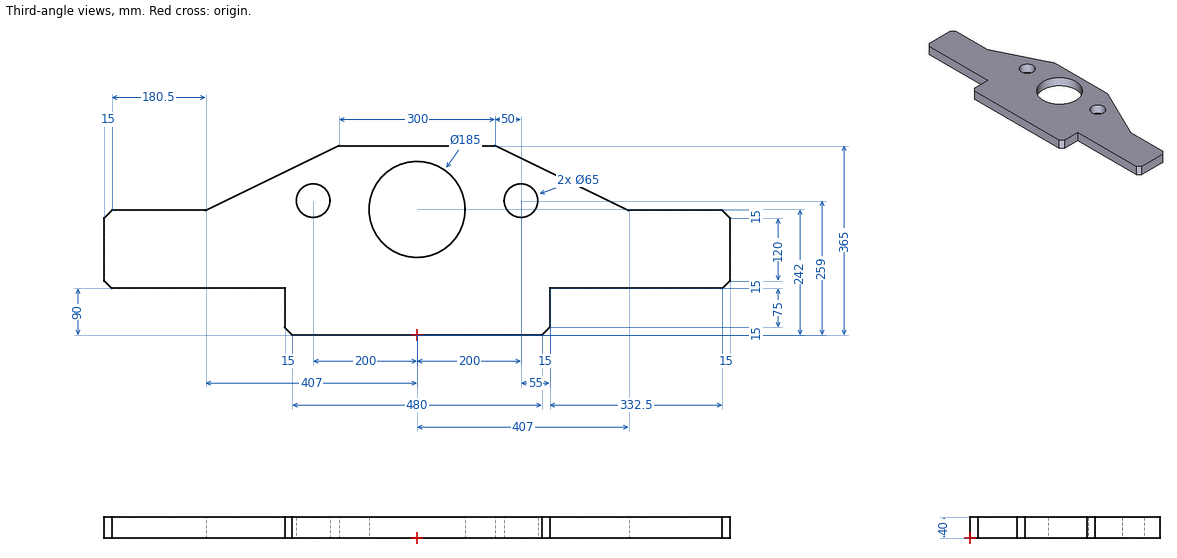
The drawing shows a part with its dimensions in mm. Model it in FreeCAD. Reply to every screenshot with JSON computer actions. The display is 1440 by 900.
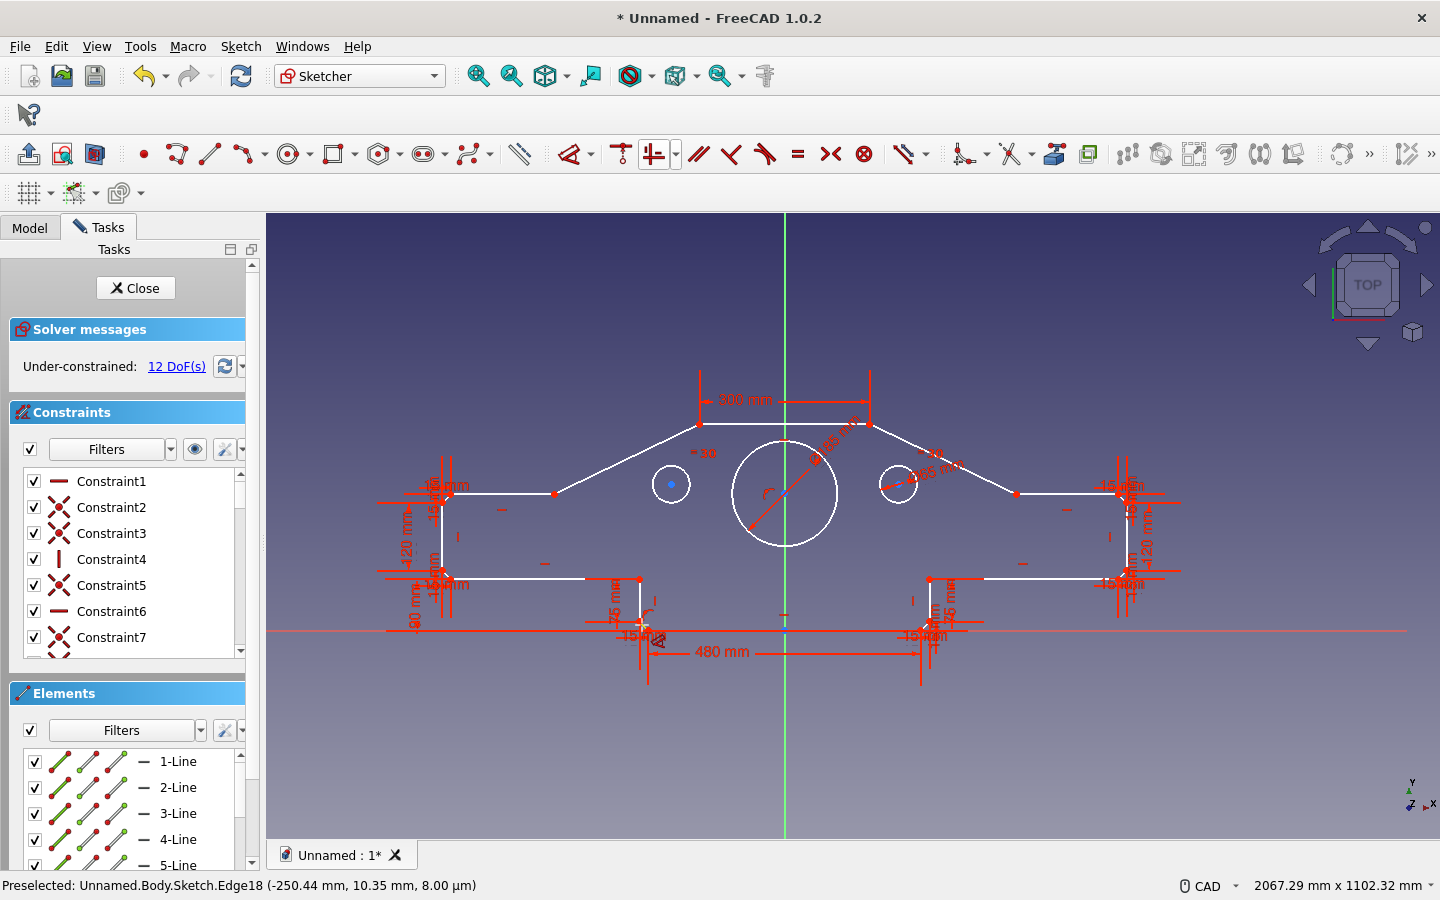
{"action": "left_click", "coordinate": [899, 484]}
{"action": "left_click", "coordinate": [842, 665]}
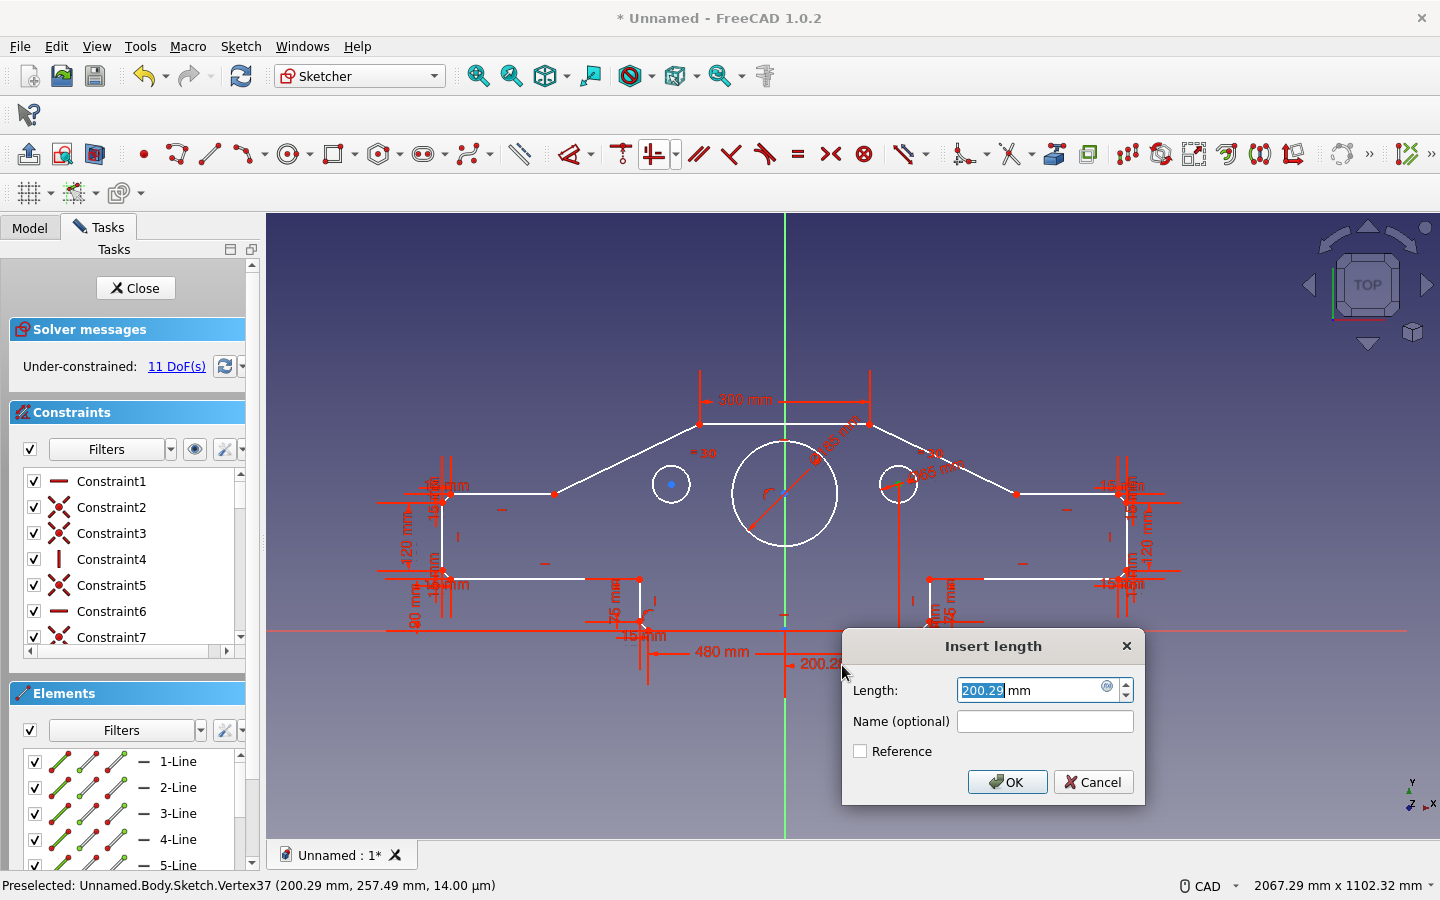
{"action": "type", "text": "200"}
{"action": "key", "text": "Return"}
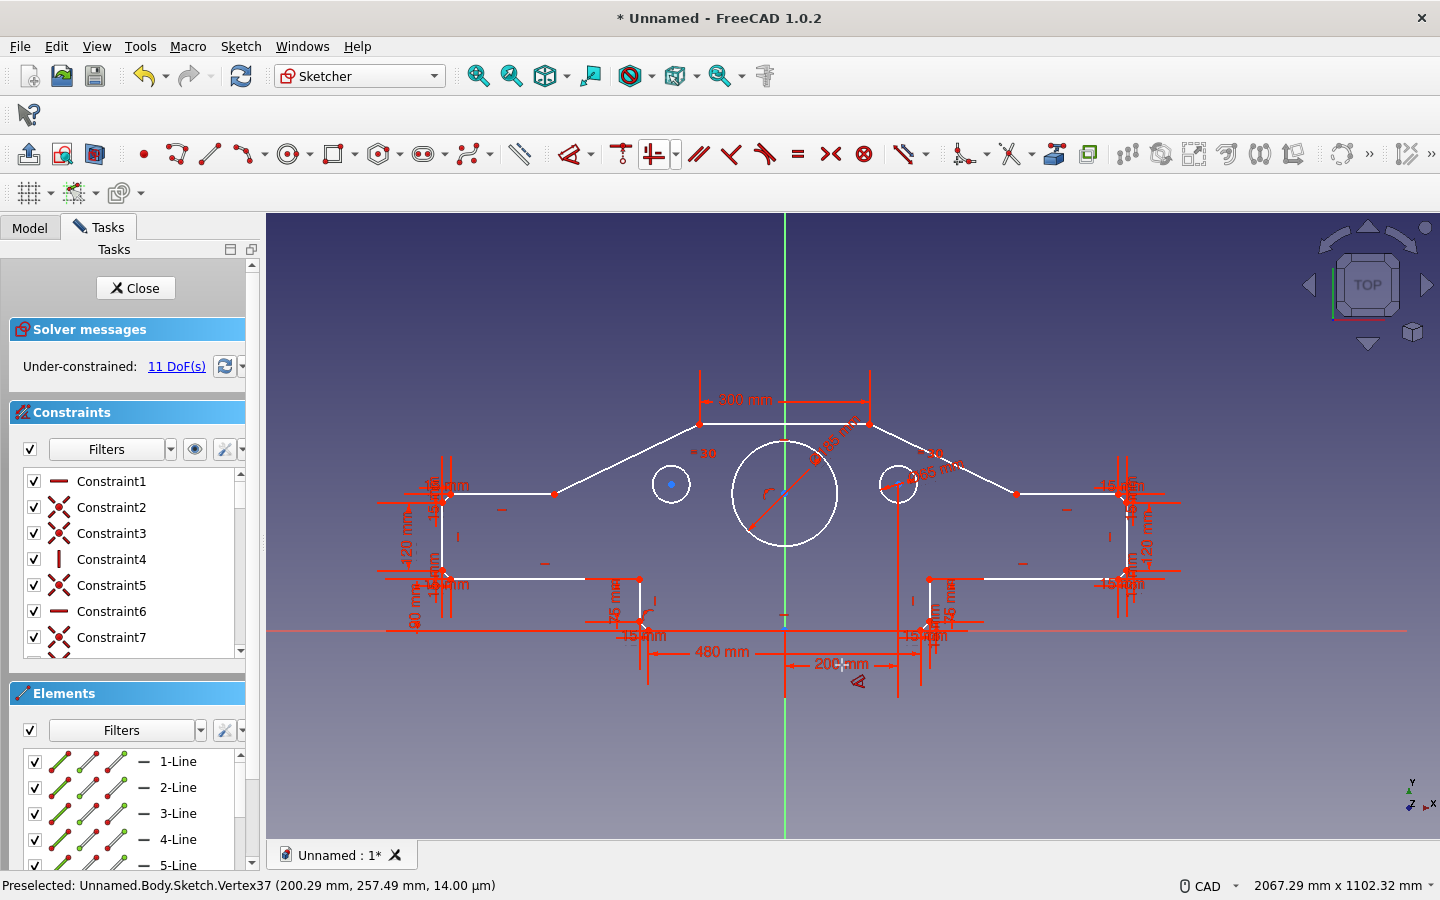
{"action": "left_click", "coordinate": [898, 484]}
{"action": "left_click", "coordinate": [932, 557]}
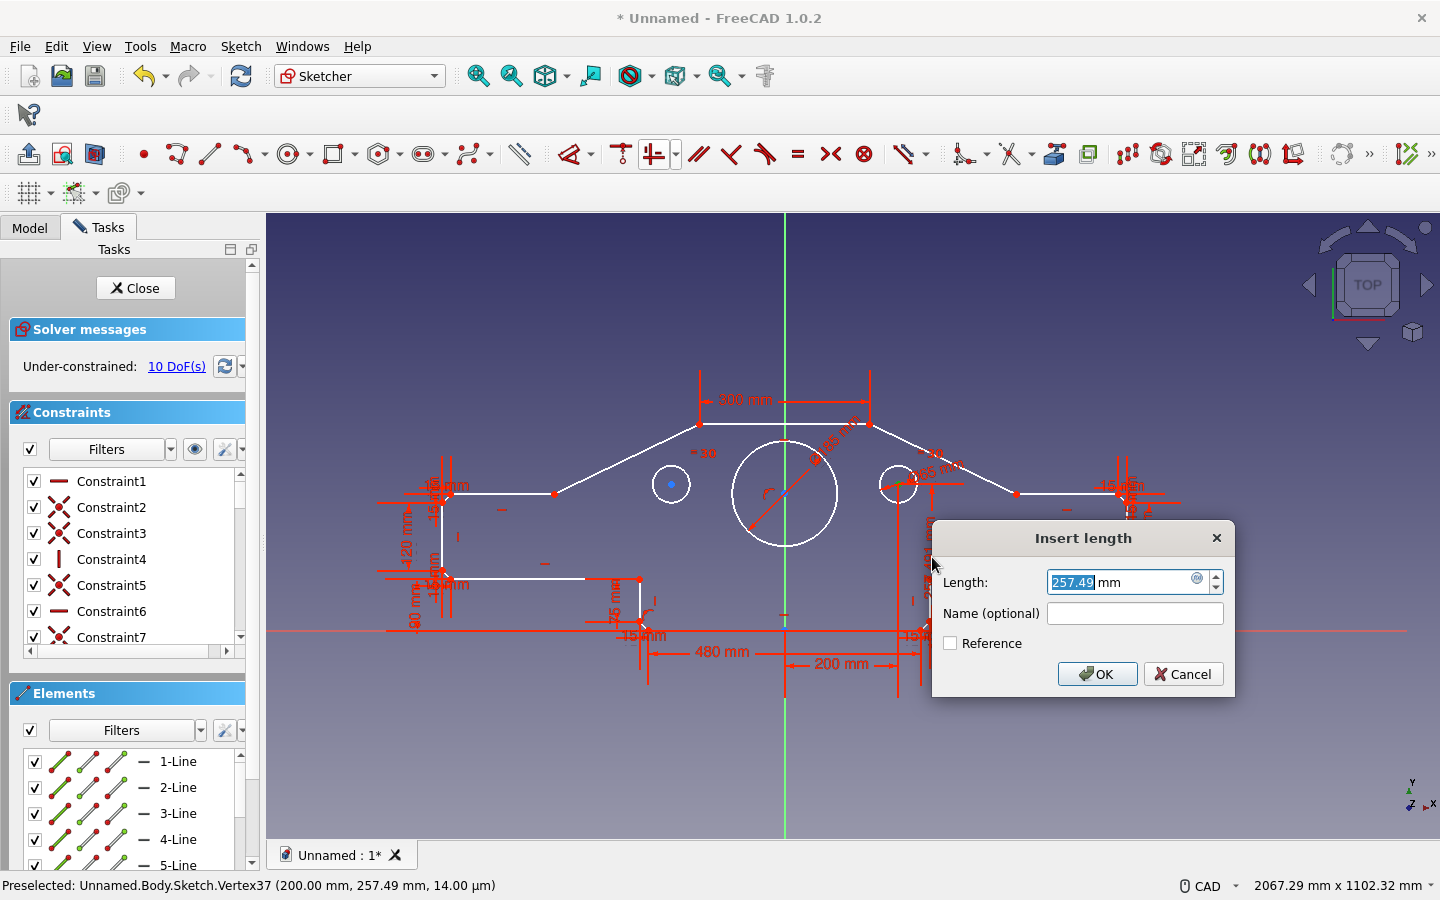
{"action": "type", "text": "259"}
{"action": "key", "text": "Return"}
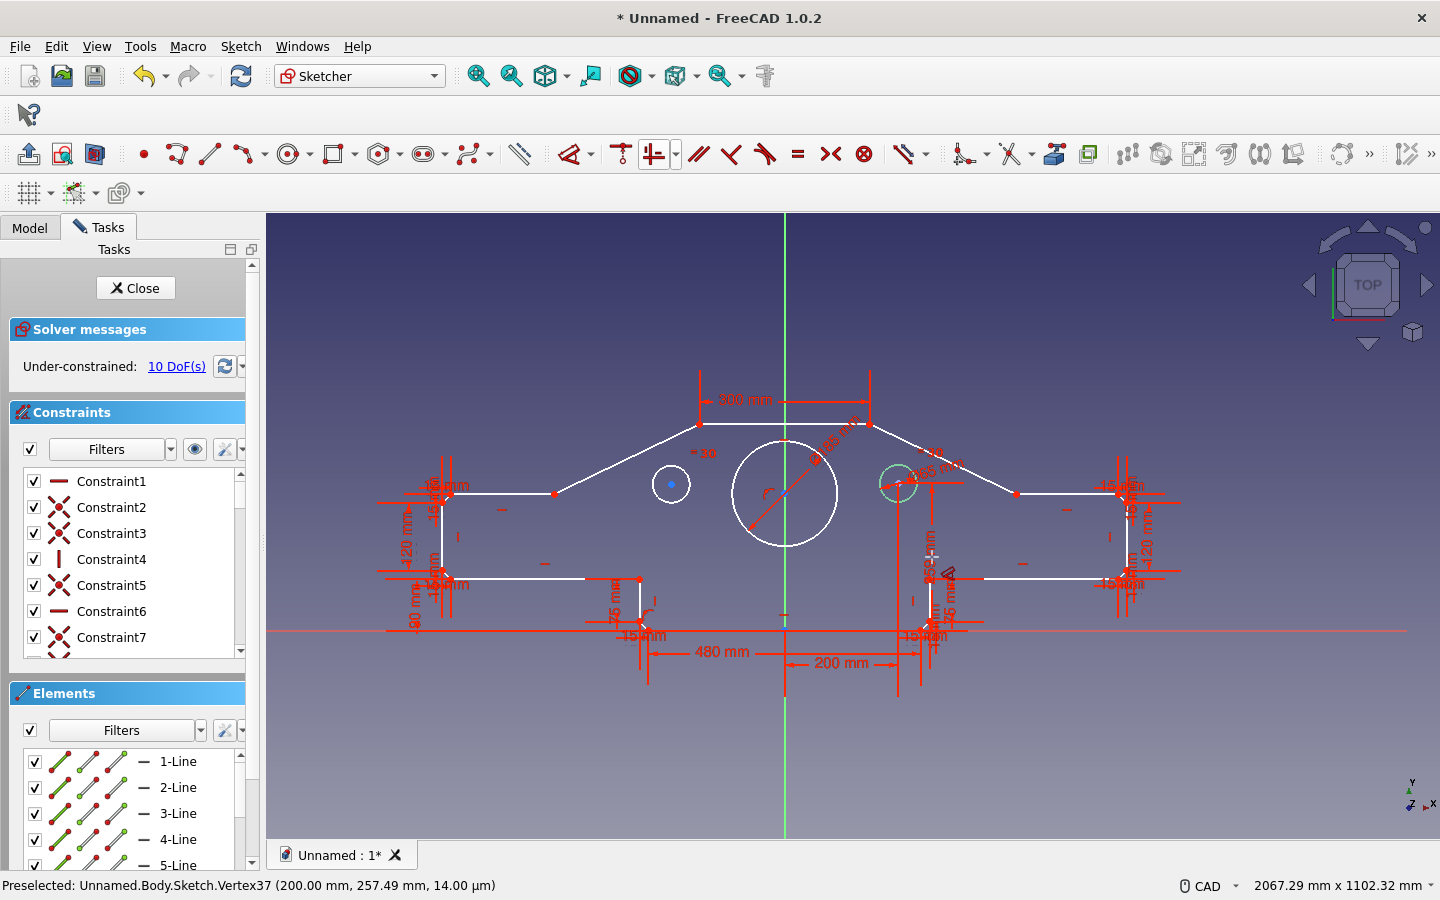
{"action": "left_click", "coordinate": [785, 494]}
{"action": "left_click", "coordinate": [819, 562]}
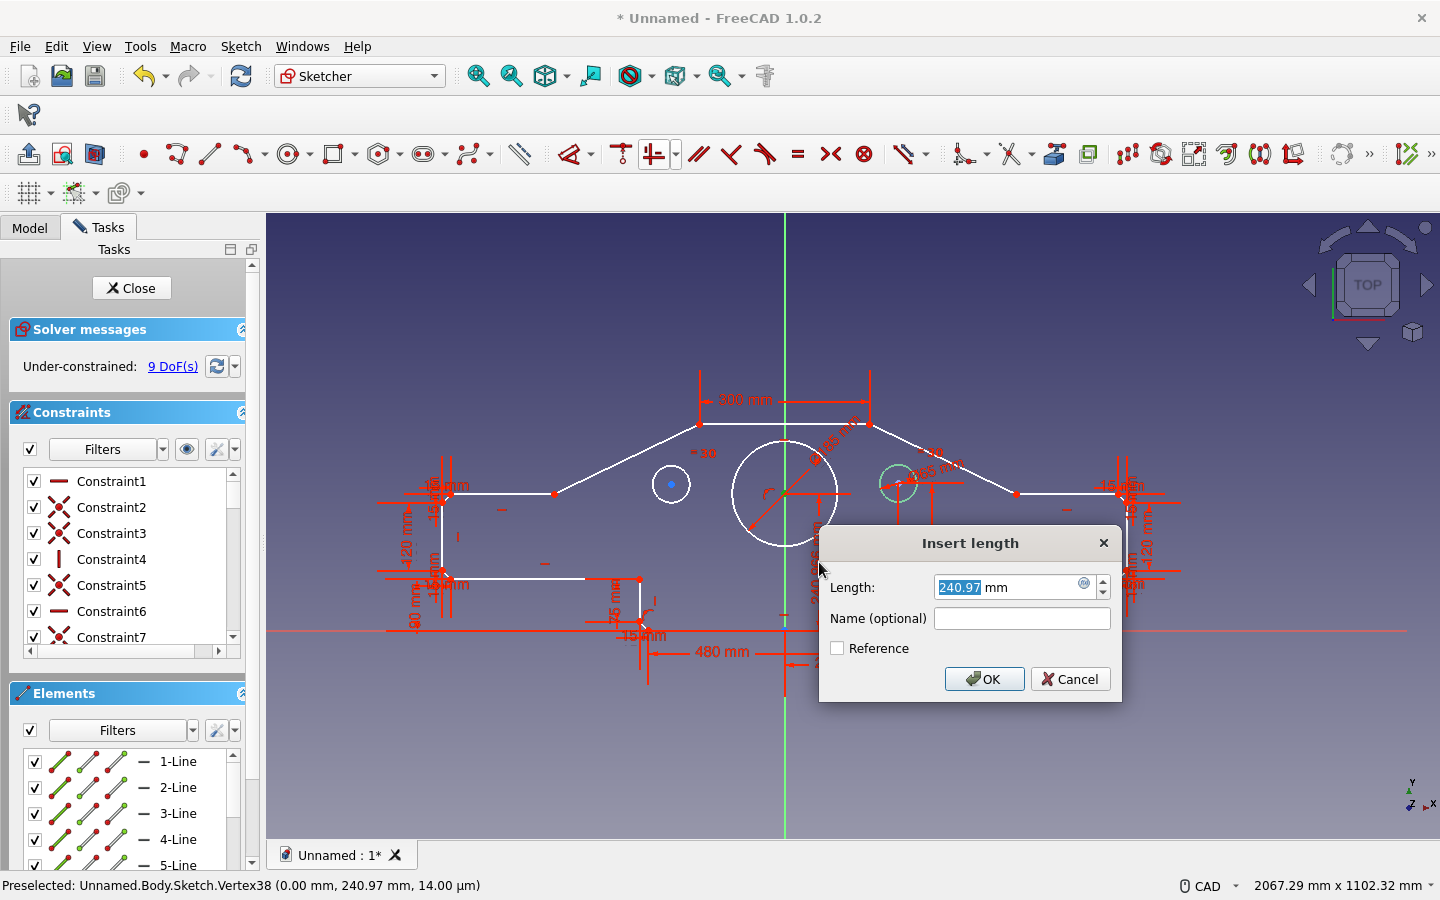
{"action": "type", "text": "242"}
{"action": "key", "text": "Return"}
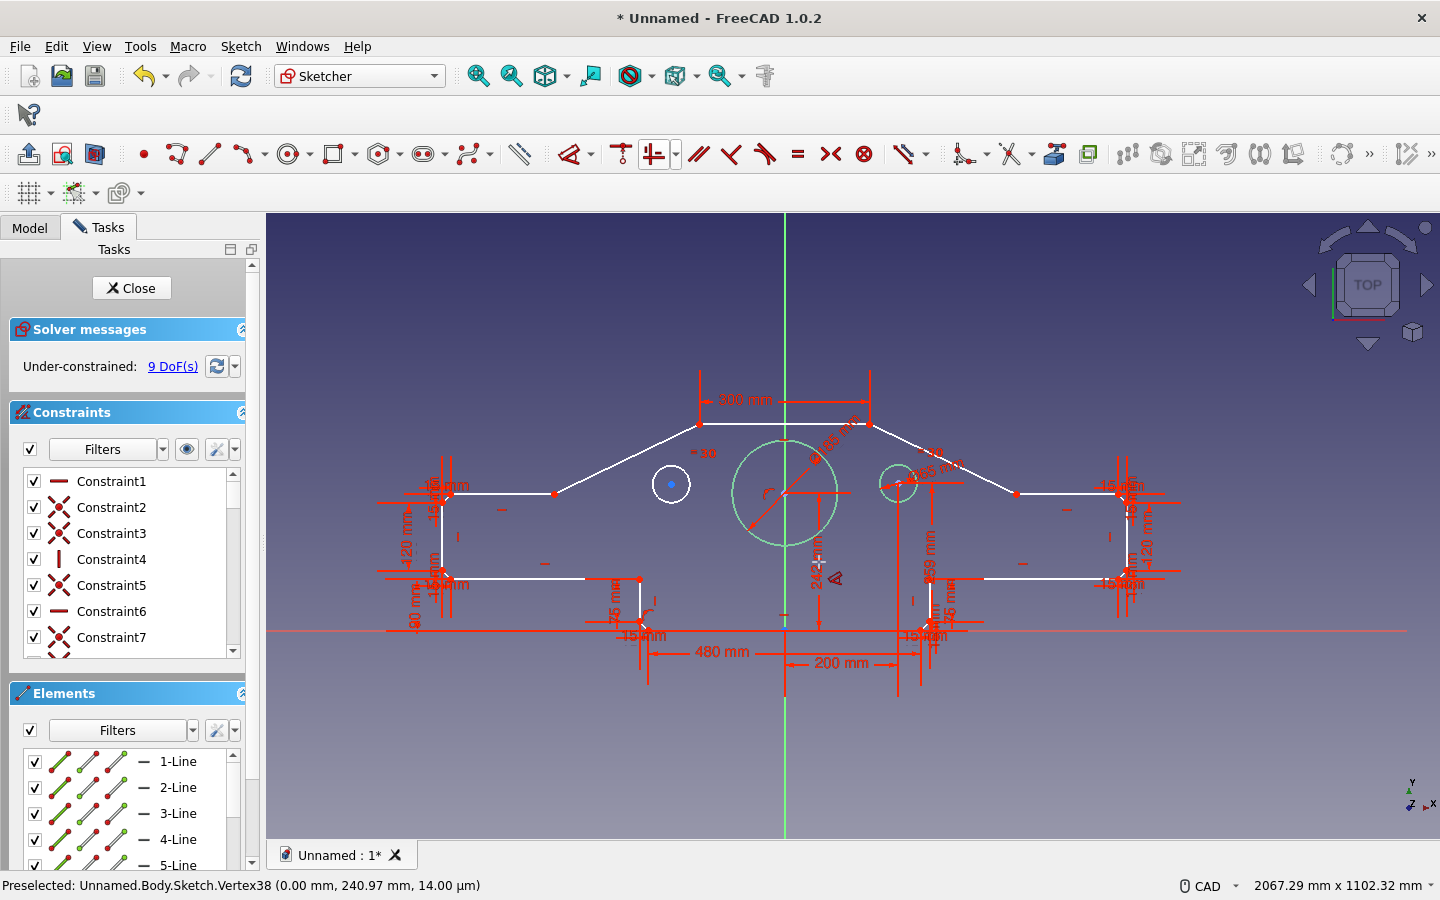
{"action": "left_click", "coordinate": [671, 484]}
{"action": "left_click", "coordinate": [728, 450]}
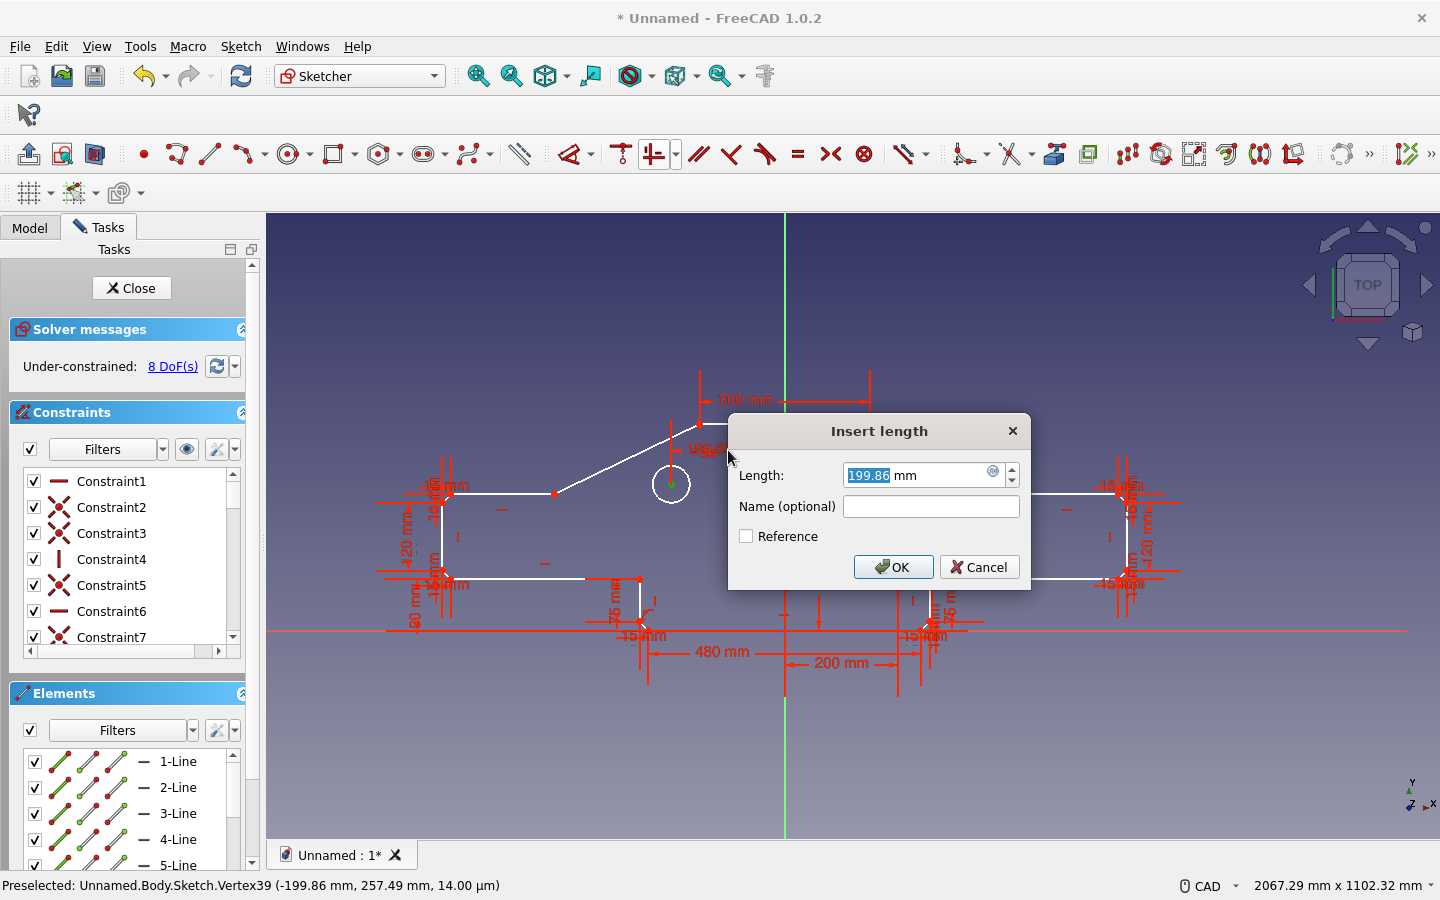
{"action": "type", "text": "200"}
{"action": "key", "text": "Return"}